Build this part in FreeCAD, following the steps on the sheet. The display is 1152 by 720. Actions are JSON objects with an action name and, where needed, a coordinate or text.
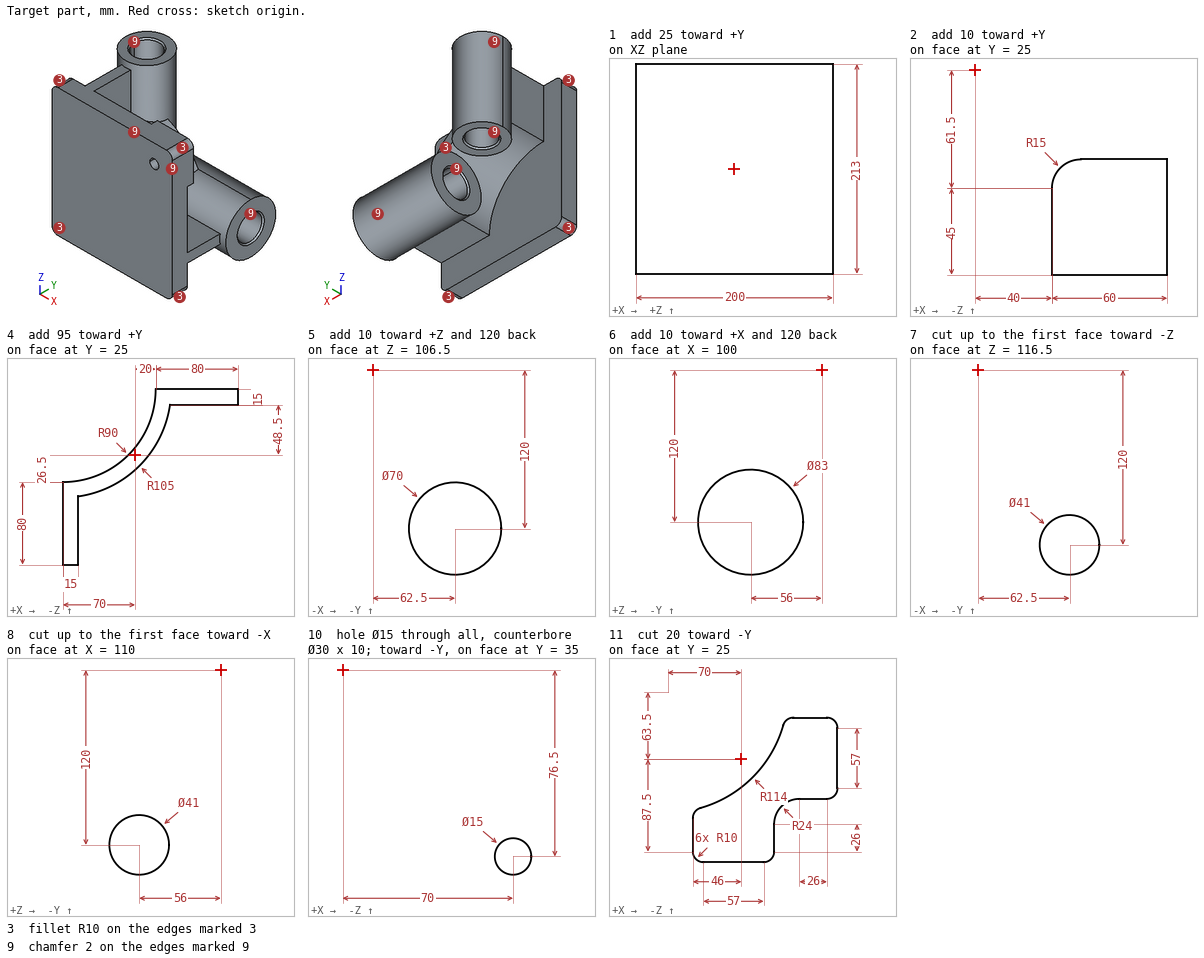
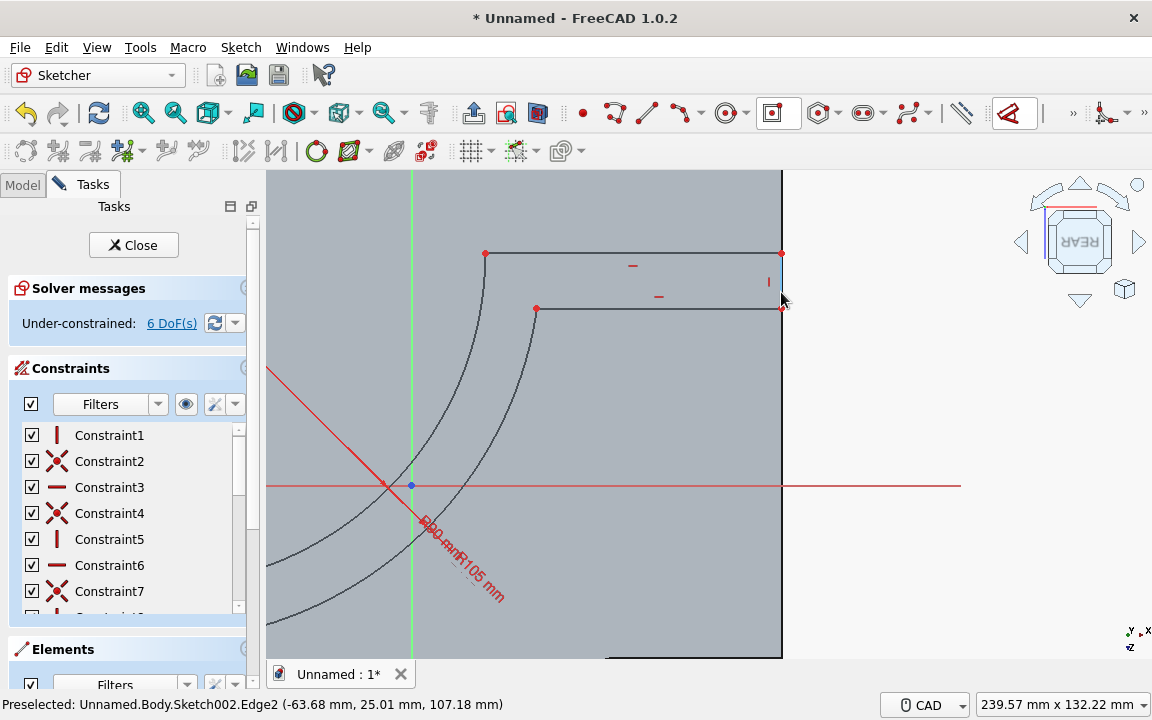
{"action": "left_click", "coordinate": [781, 292]}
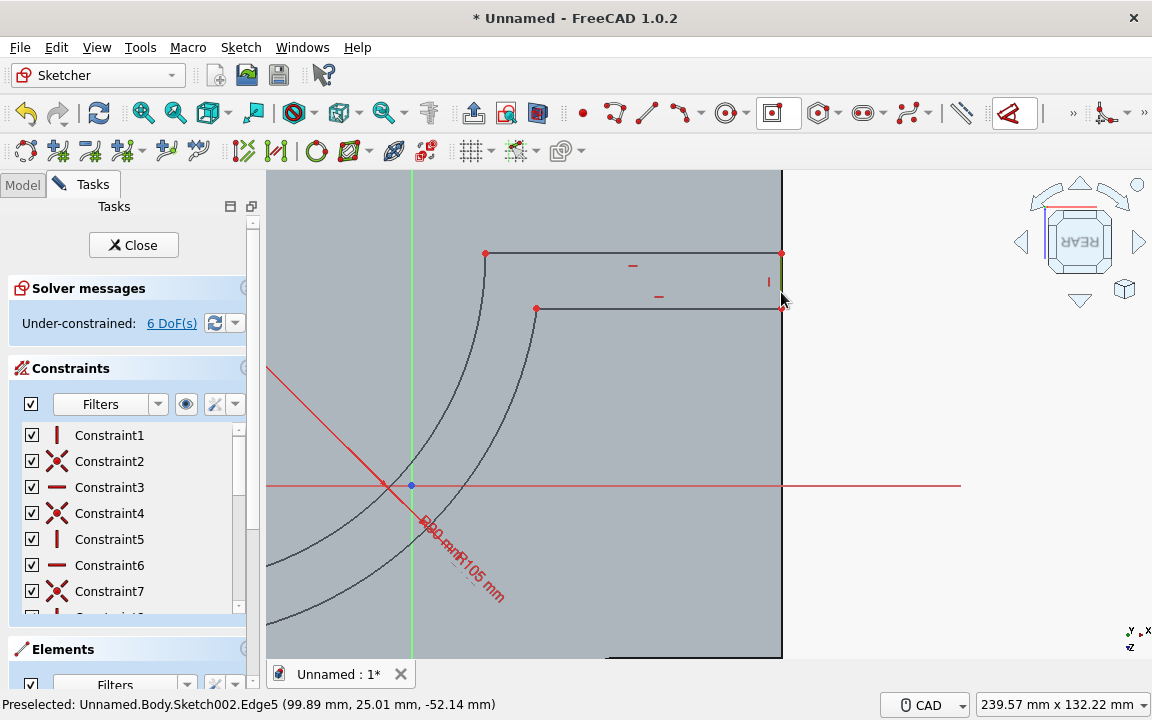
{"action": "left_click", "coordinate": [1032, 114]}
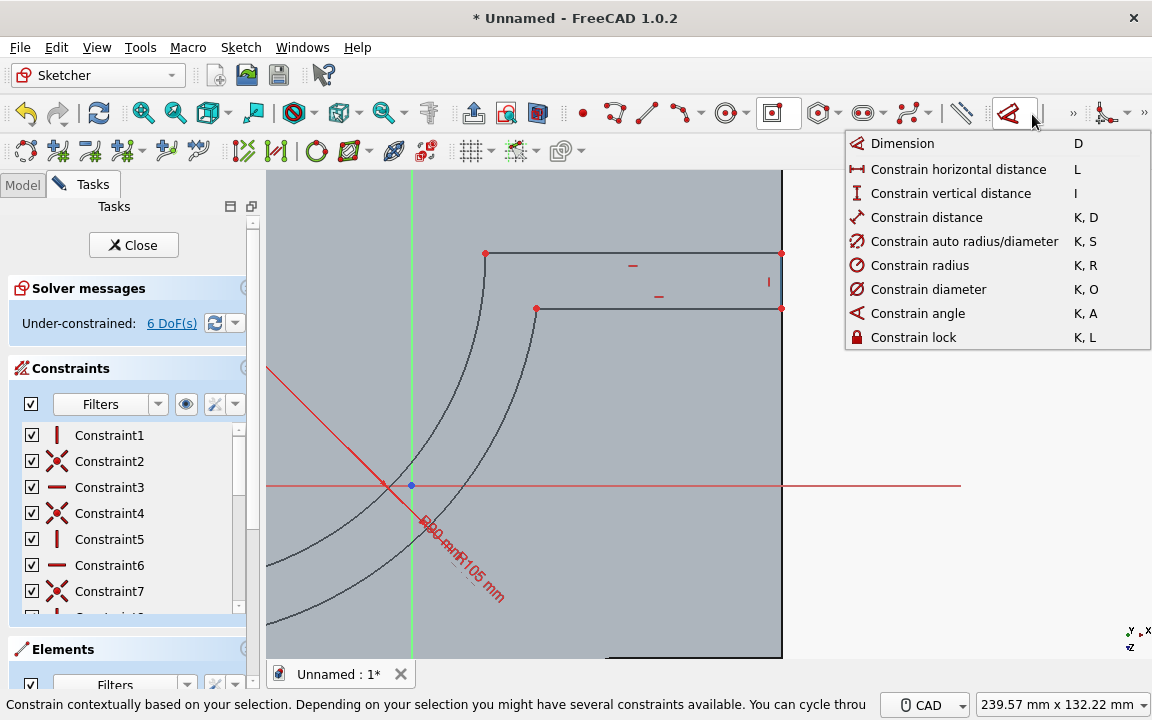
{"action": "left_click", "coordinate": [998, 193]}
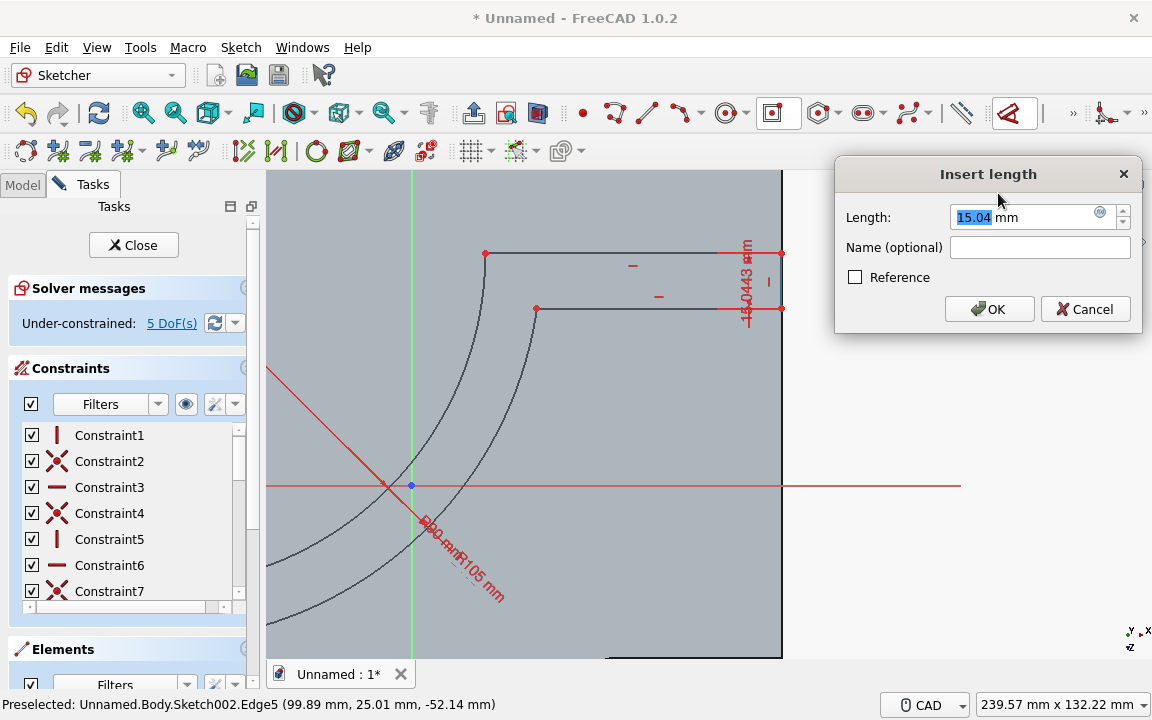
{"action": "type", "text": "15"}
{"action": "key", "text": "Return"}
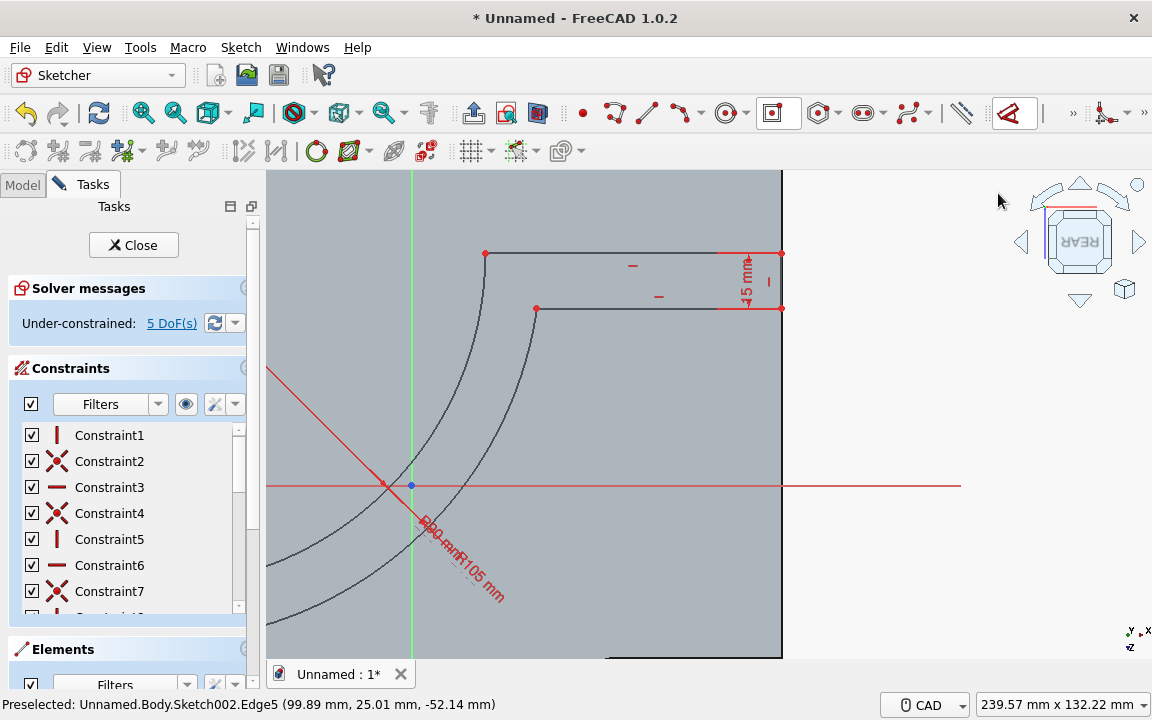
{"action": "left_click", "coordinate": [693, 253]}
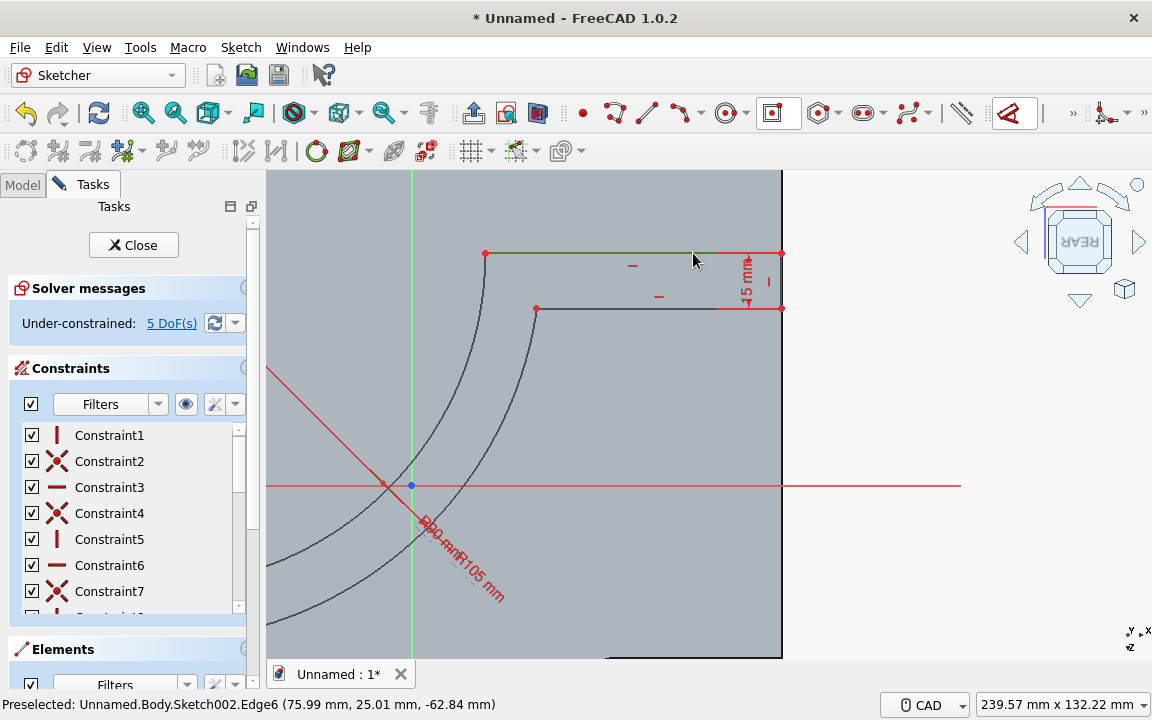
{"action": "left_click", "coordinate": [1032, 114]}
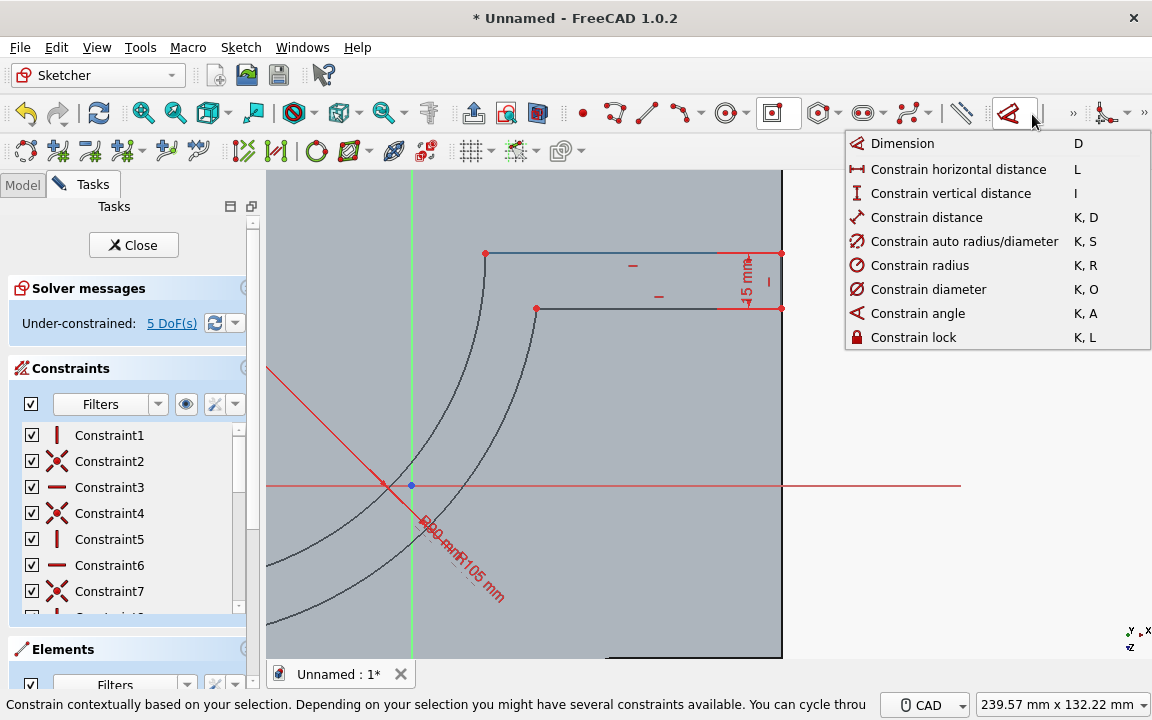
{"action": "left_click", "coordinate": [998, 169]}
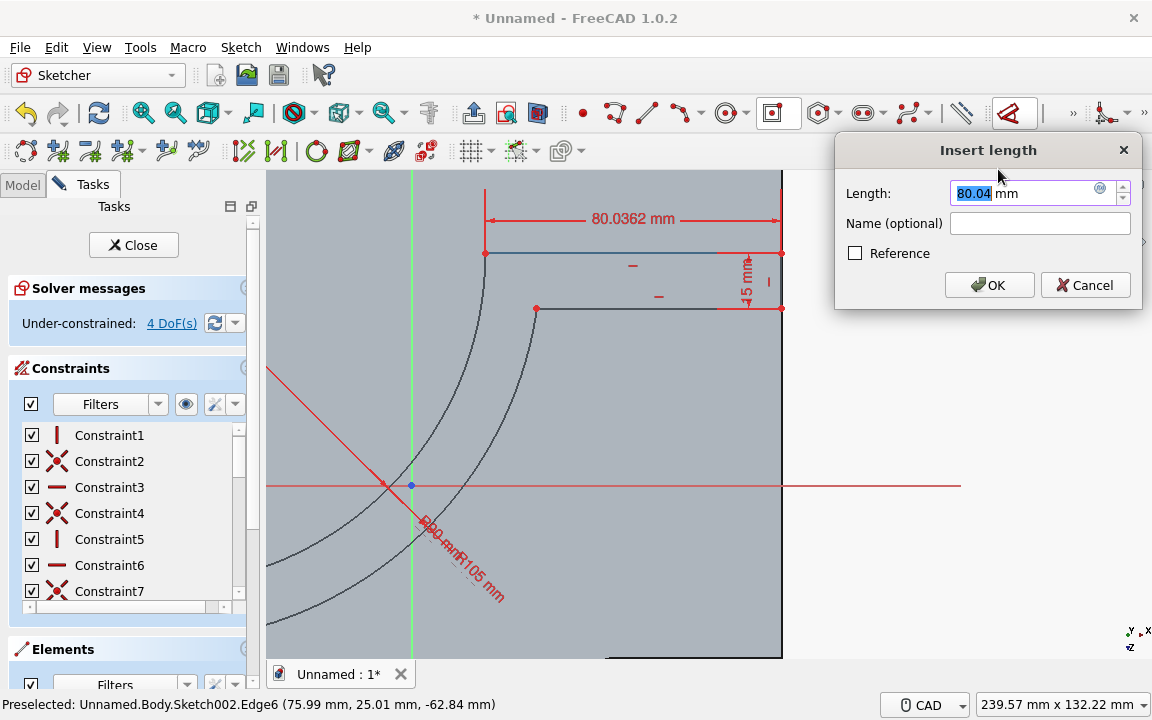
{"action": "type", "text": "80"}
{"action": "key", "text": "Return"}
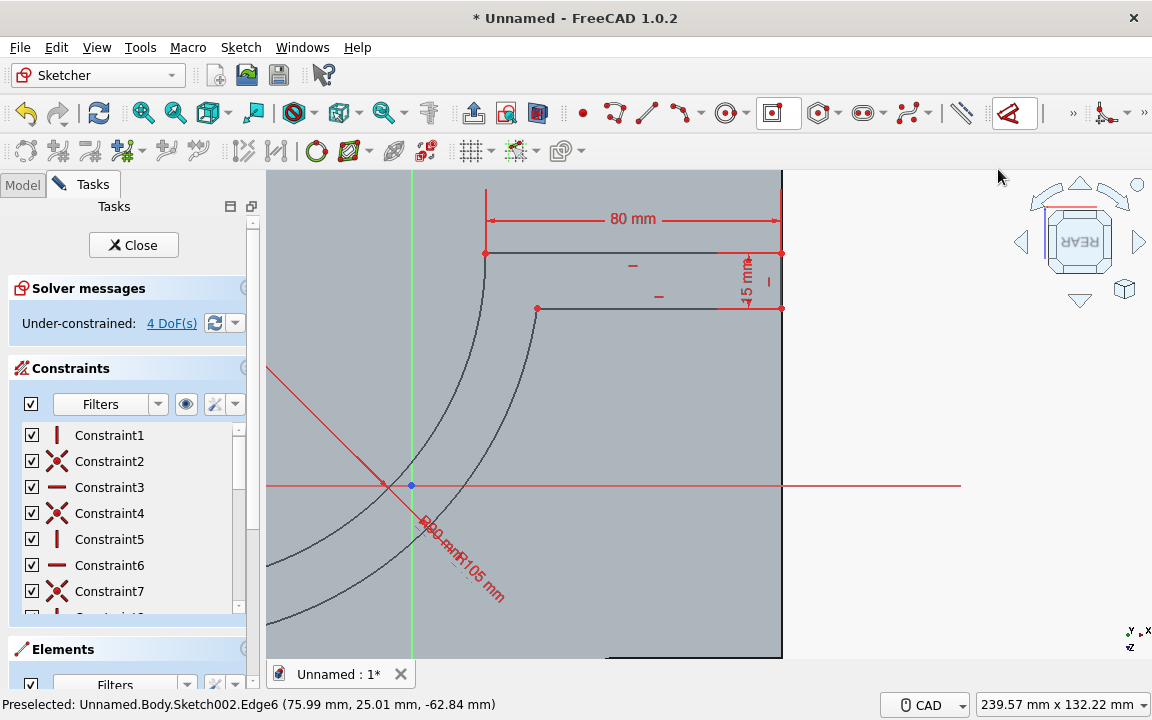
{"action": "scroll", "coordinate": [782, 291], "scroll_direction": "down", "scroll_amount": 4}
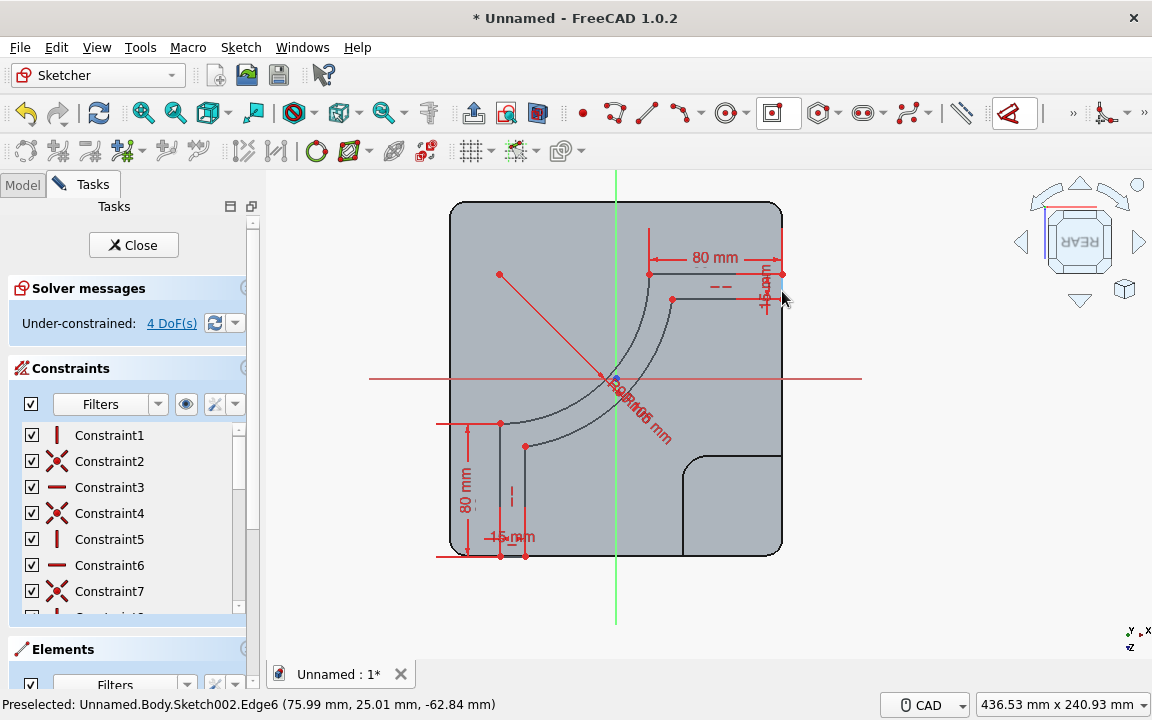
{"action": "left_click", "coordinate": [500, 424]}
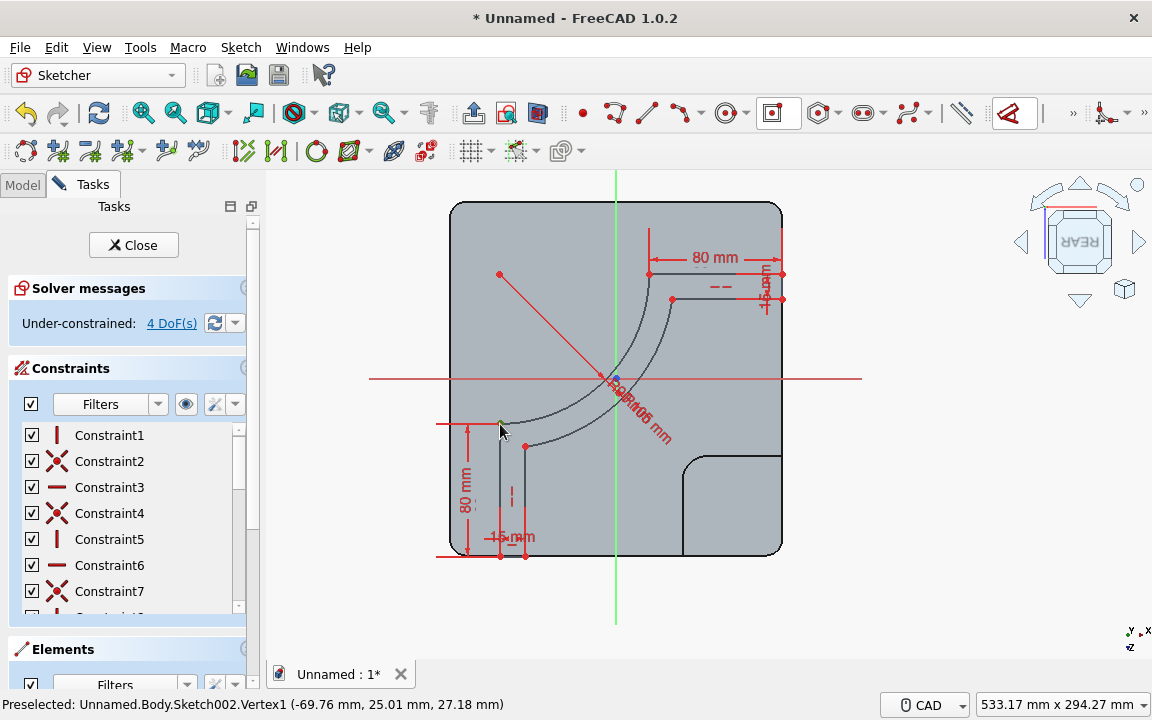
{"action": "key", "text": "l"}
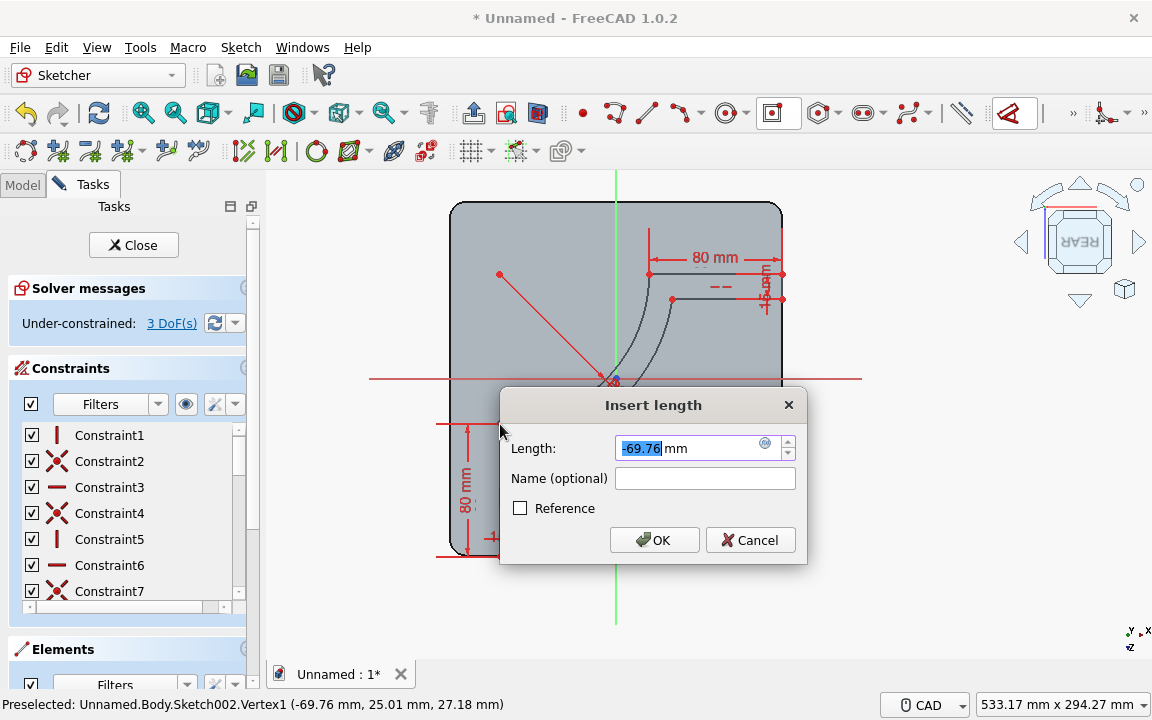
{"action": "type", "text": "-70"}
{"action": "key", "text": "Return"}